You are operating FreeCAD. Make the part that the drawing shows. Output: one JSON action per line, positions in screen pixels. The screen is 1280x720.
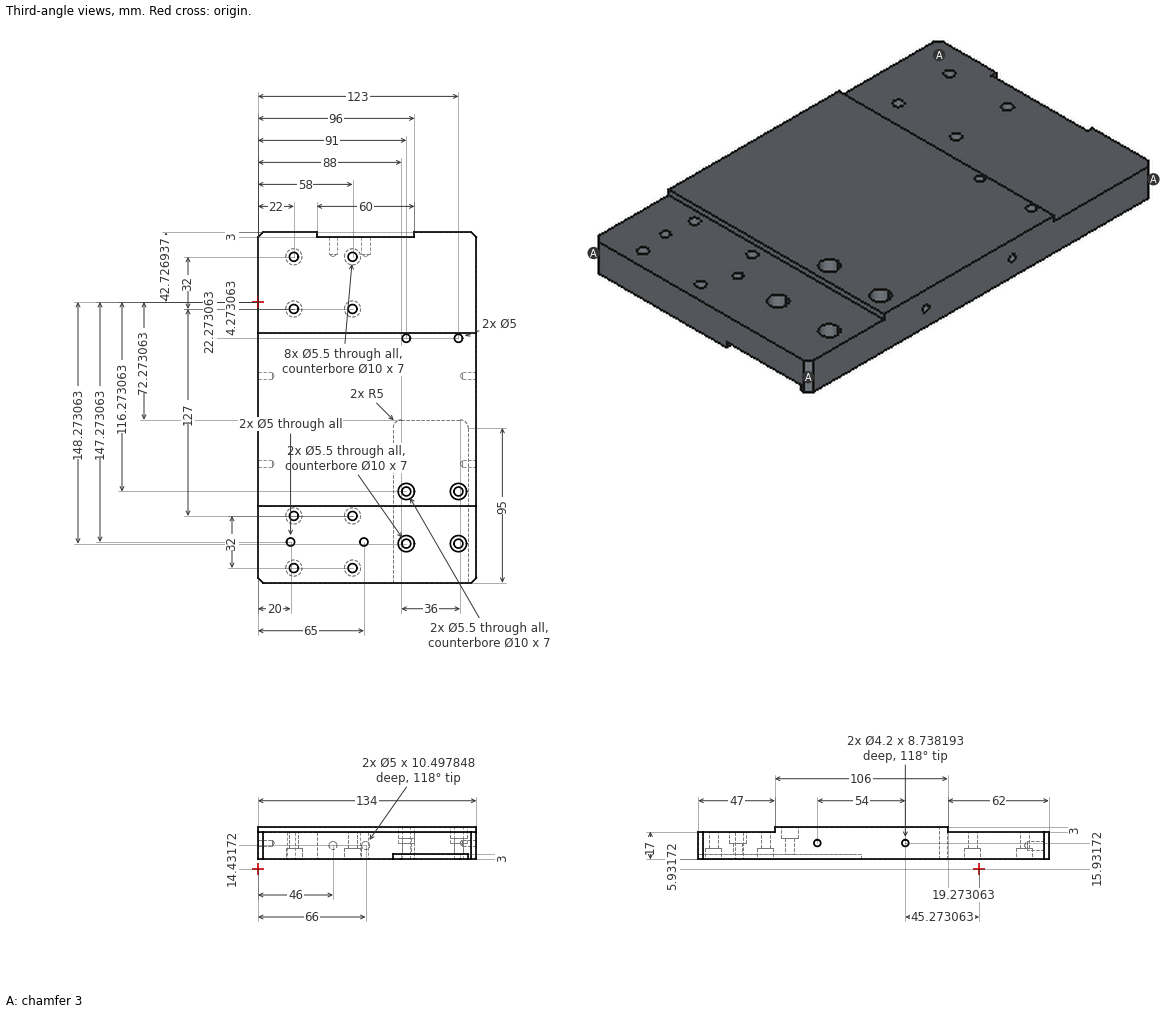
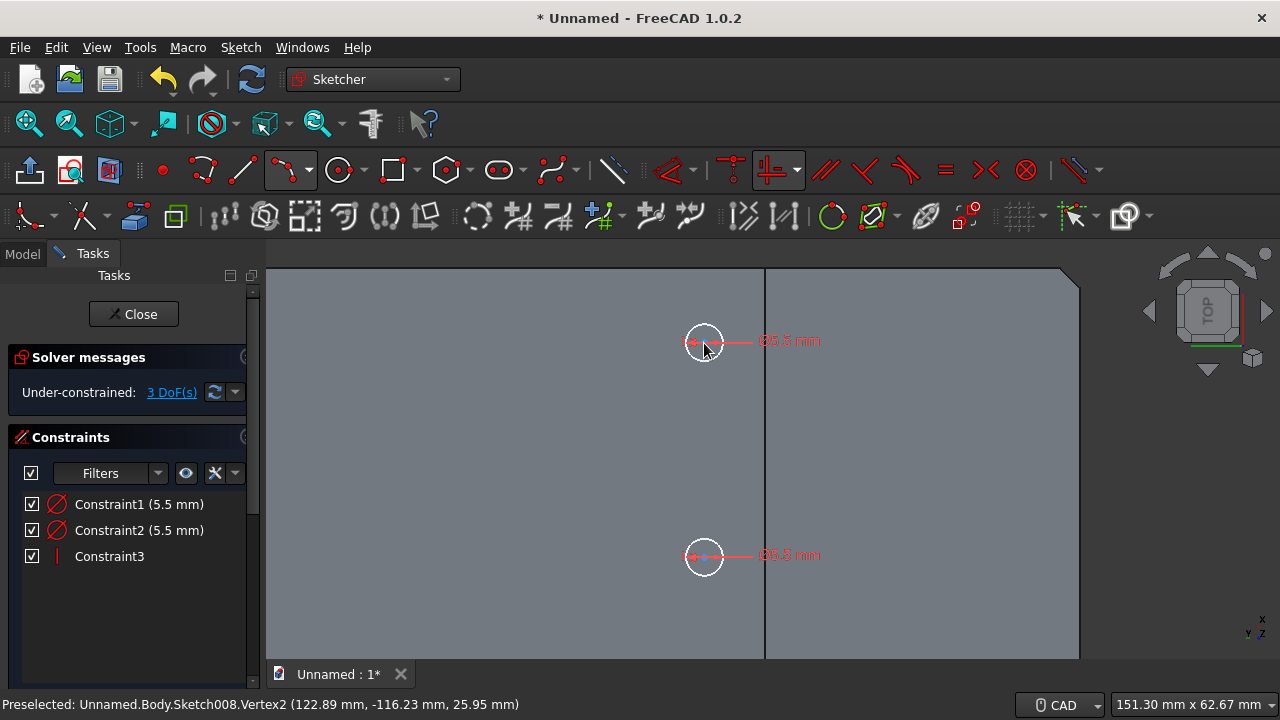
{"action": "left_click", "coordinate": [668, 170]}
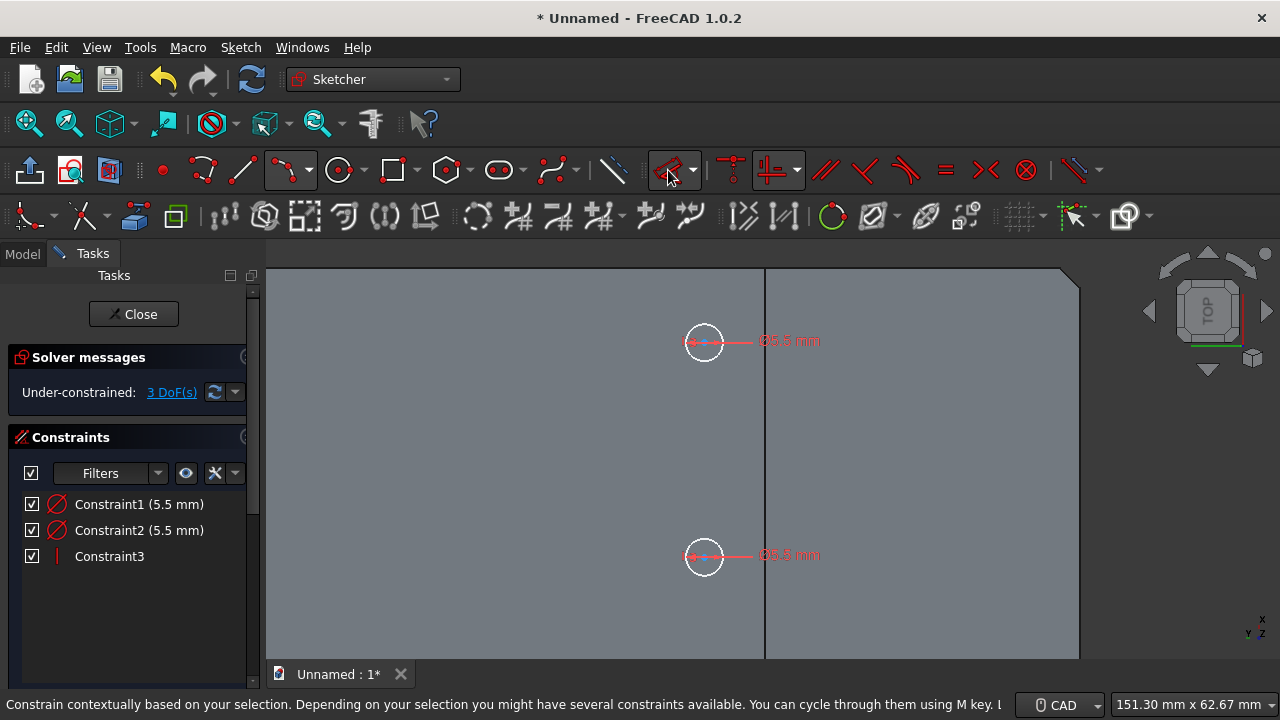
{"action": "left_click", "coordinate": [704, 557]}
{"action": "left_click", "coordinate": [738, 594]}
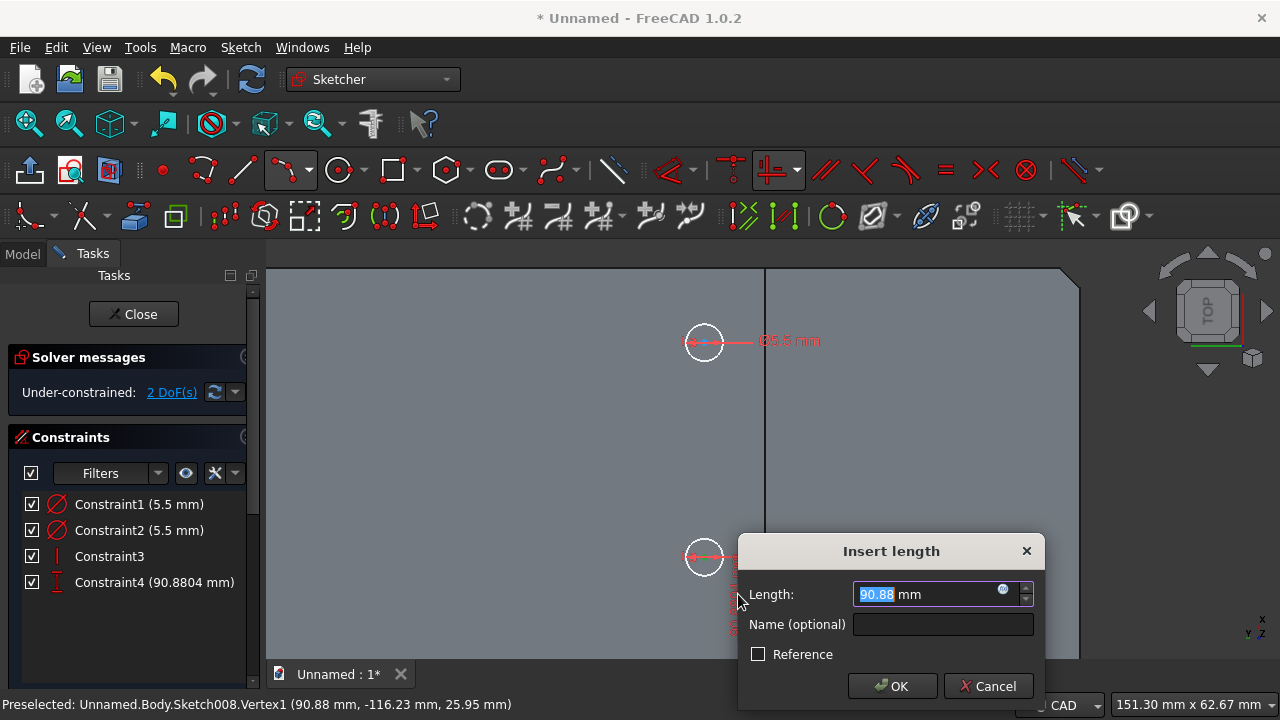
{"action": "type", "text": "91"}
{"action": "key", "text": "Return"}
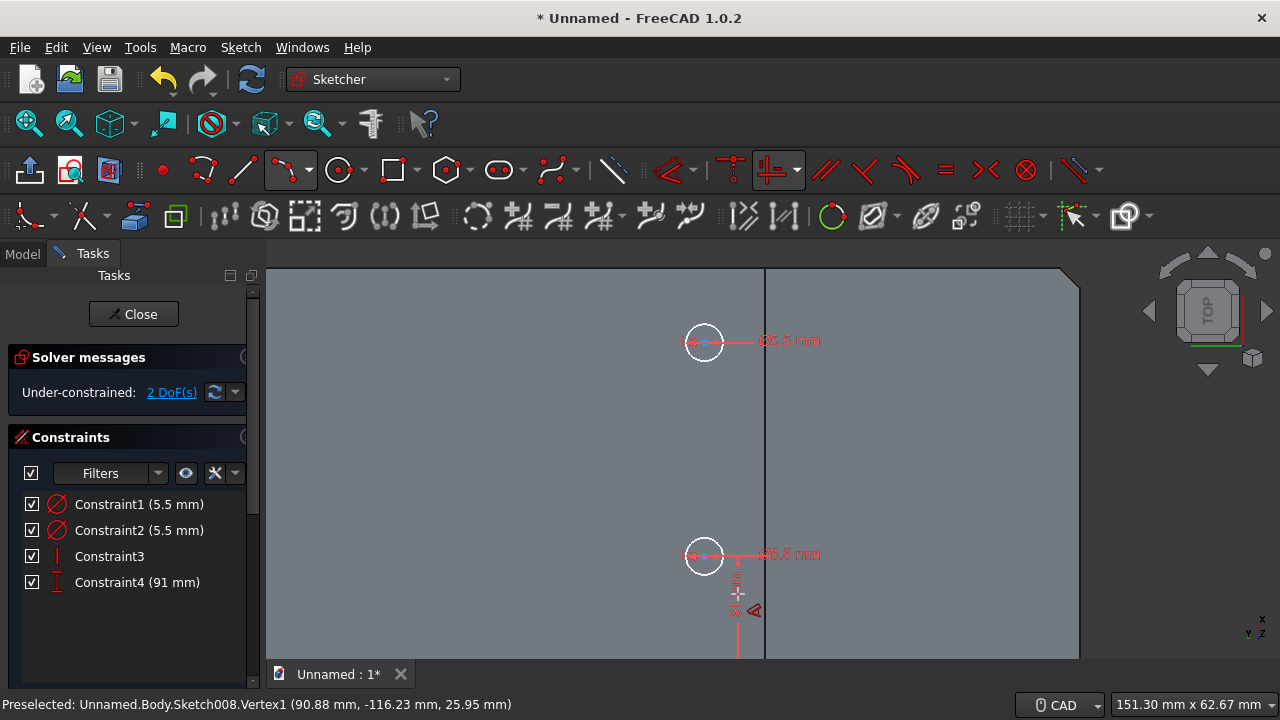
{"action": "left_click", "coordinate": [704, 343]}
{"action": "left_click", "coordinate": [738, 487]}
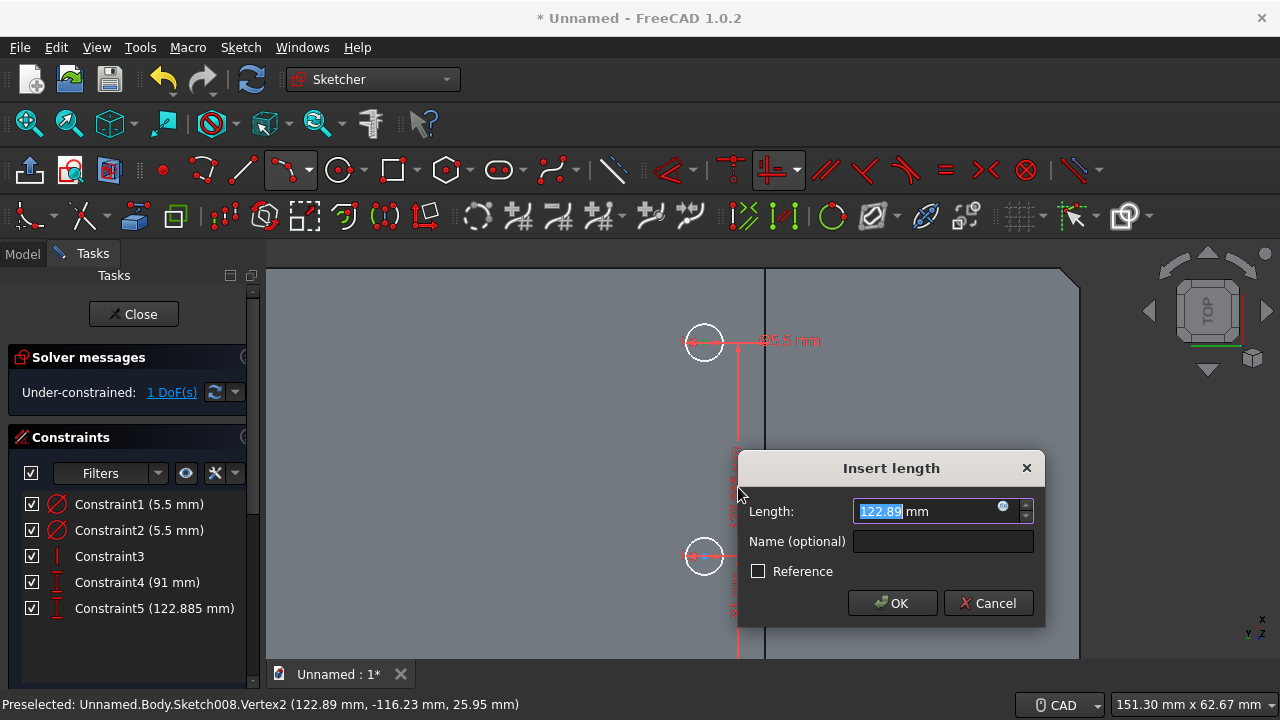
{"action": "type", "text": "123"}
{"action": "key", "text": "Return"}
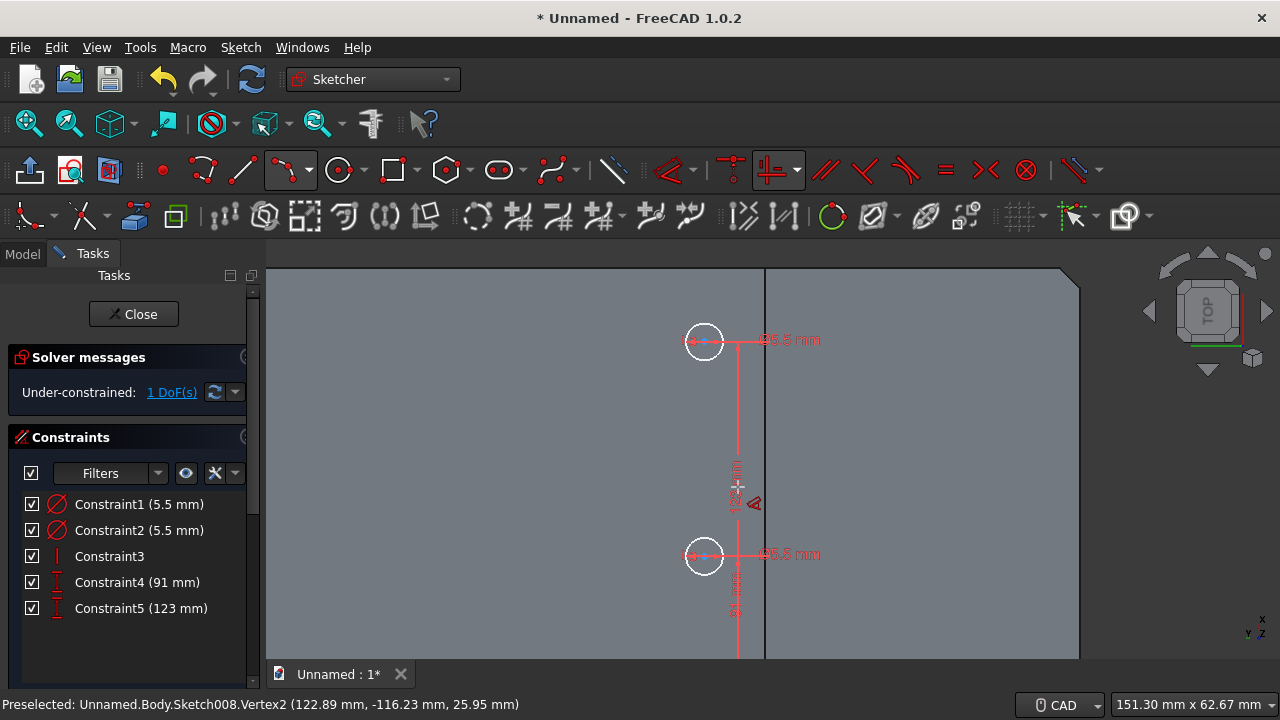
{"action": "left_click", "coordinate": [704, 556]}
{"action": "left_click", "coordinate": [499, 522]}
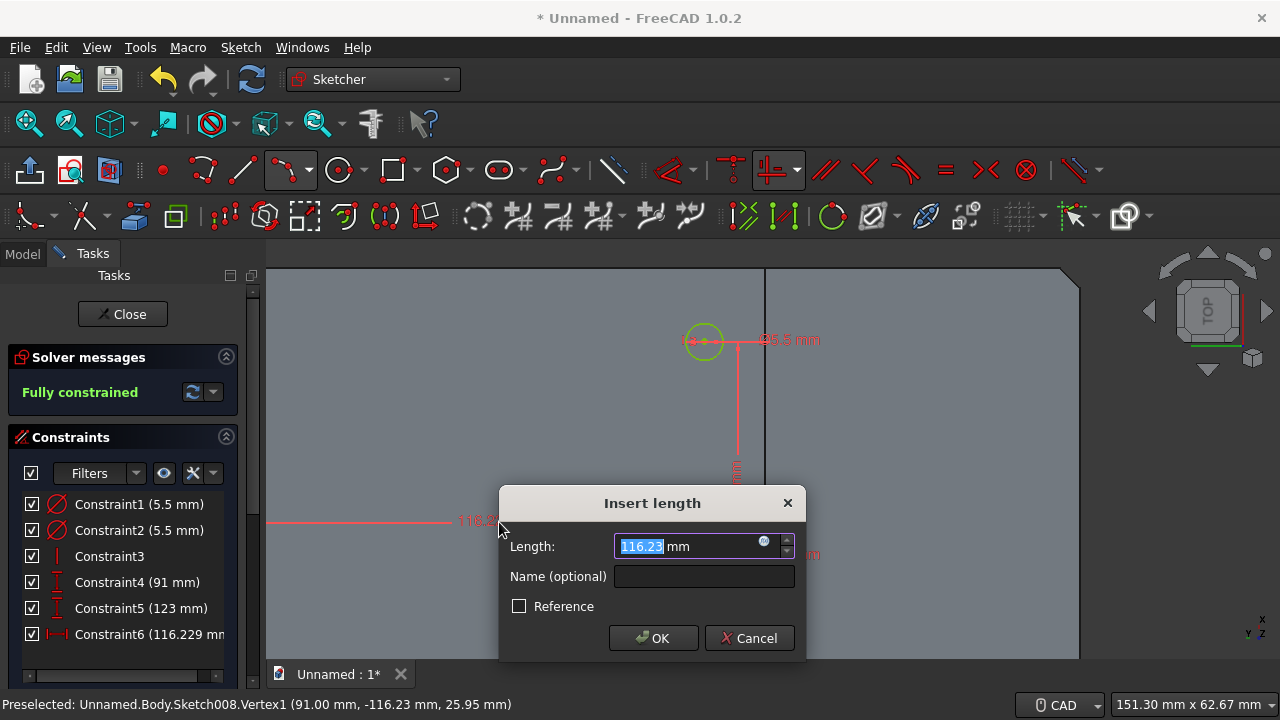
{"action": "type", "text": "116.273063"}
{"action": "key", "text": "Return"}
{"action": "key", "text": "Escape"}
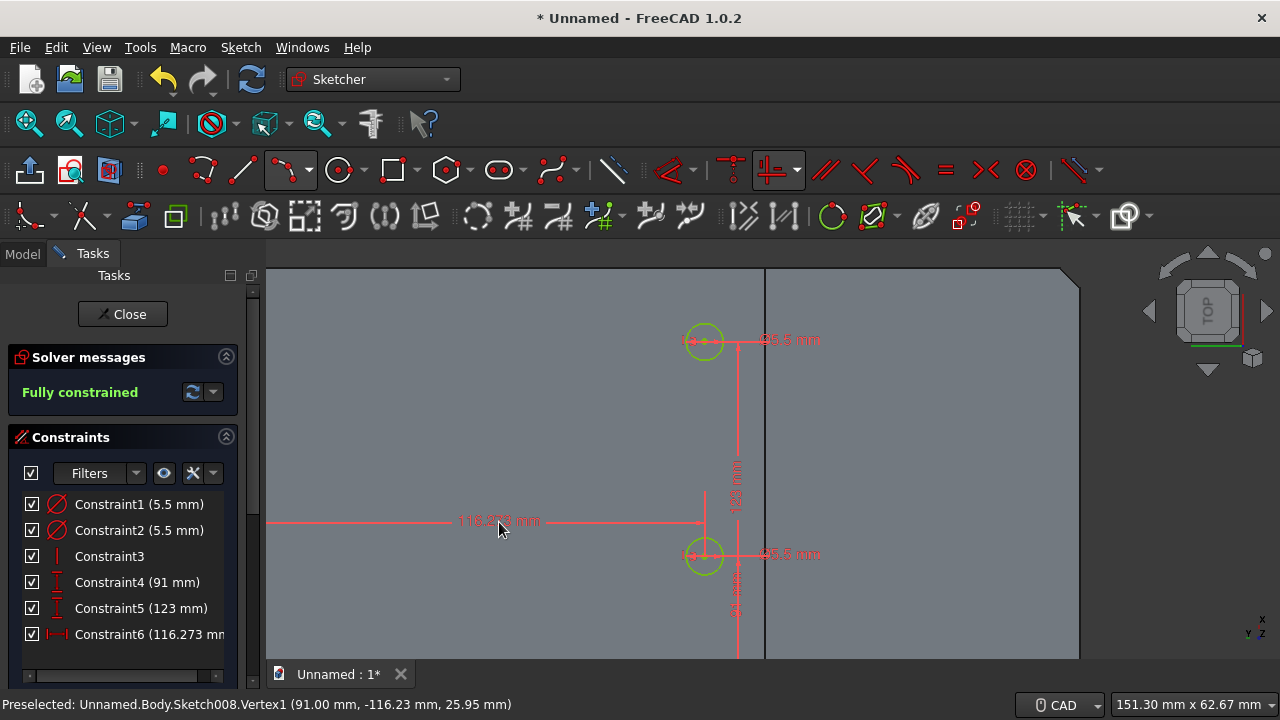
{"action": "left_click", "coordinate": [123, 314]}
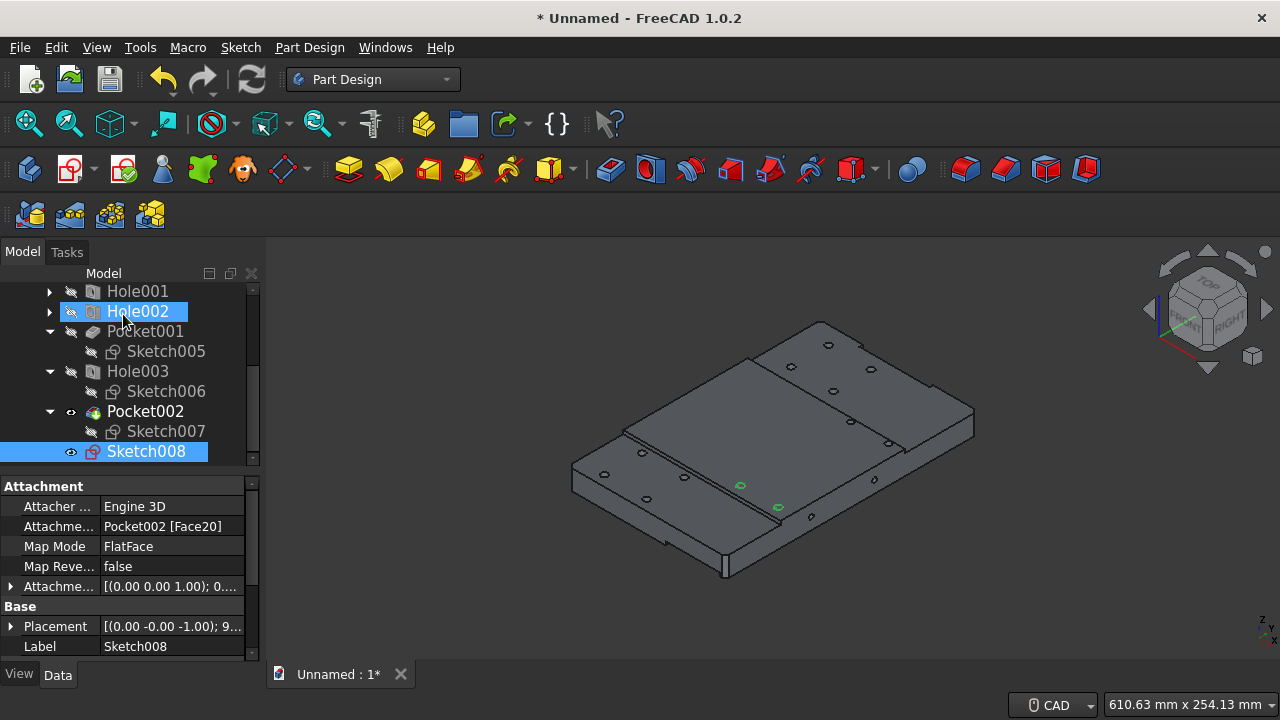
{"action": "left_click", "coordinate": [652, 170]}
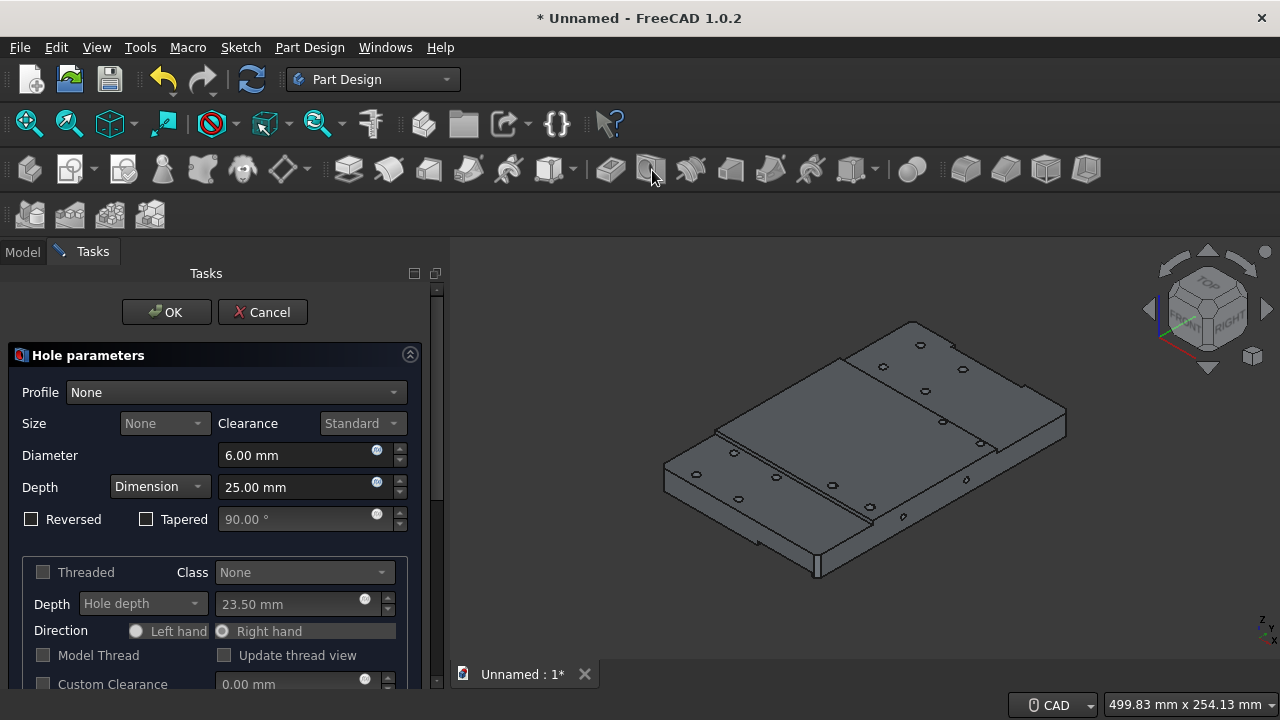
{"action": "triple_click", "coordinate": [305, 455]}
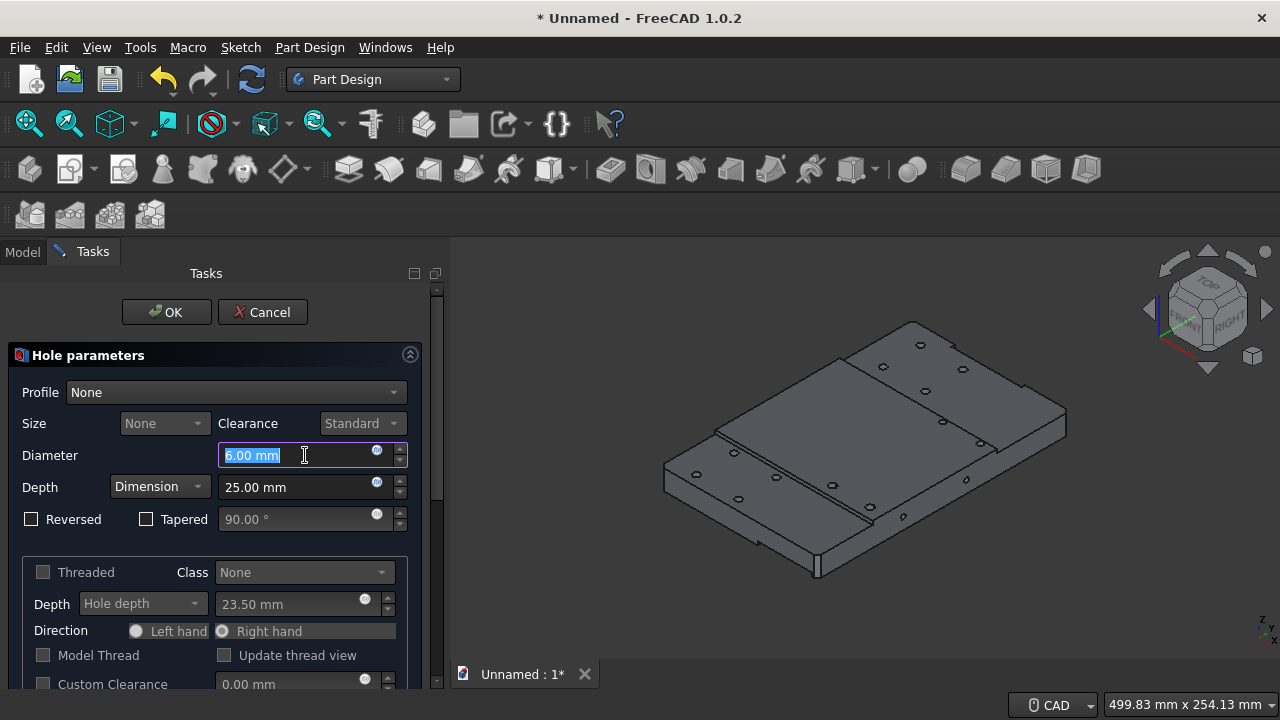
{"action": "type", "text": "5.5"}
{"action": "key", "text": "Tab"}